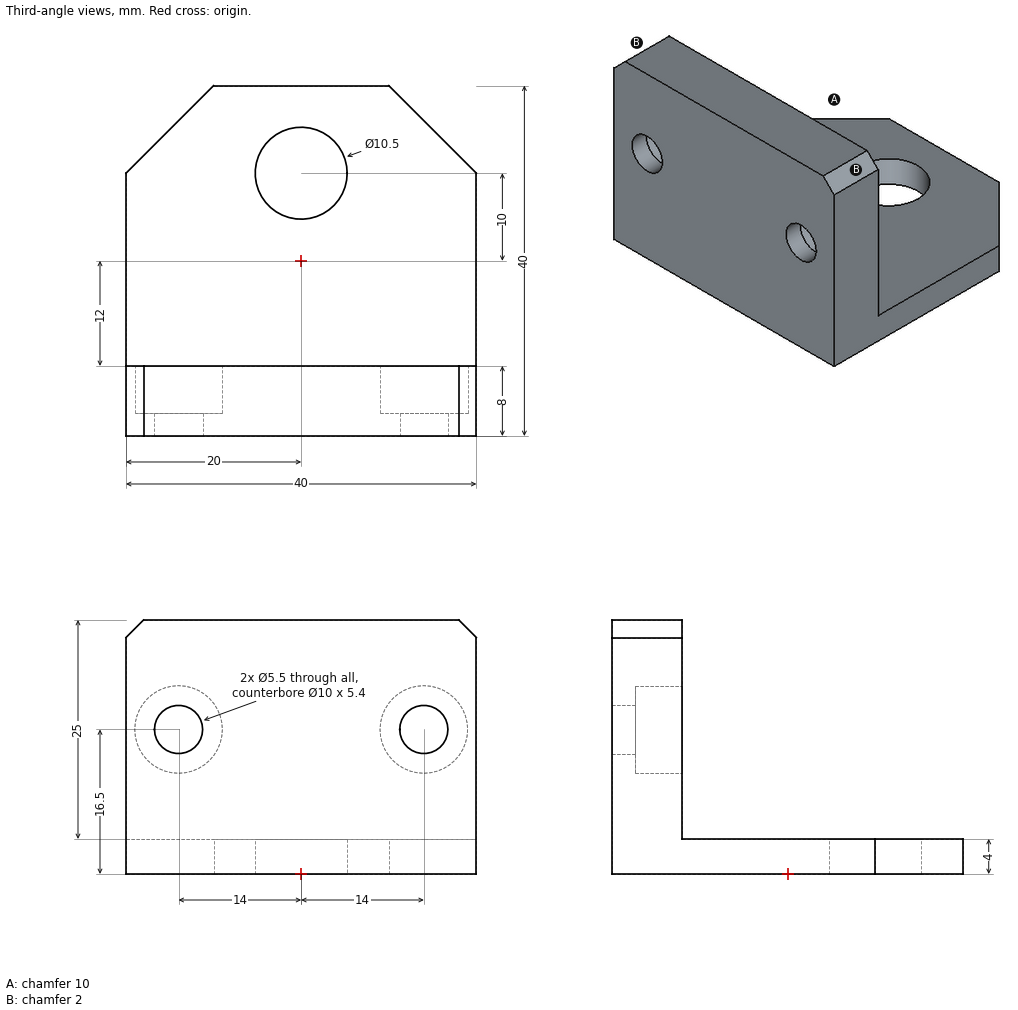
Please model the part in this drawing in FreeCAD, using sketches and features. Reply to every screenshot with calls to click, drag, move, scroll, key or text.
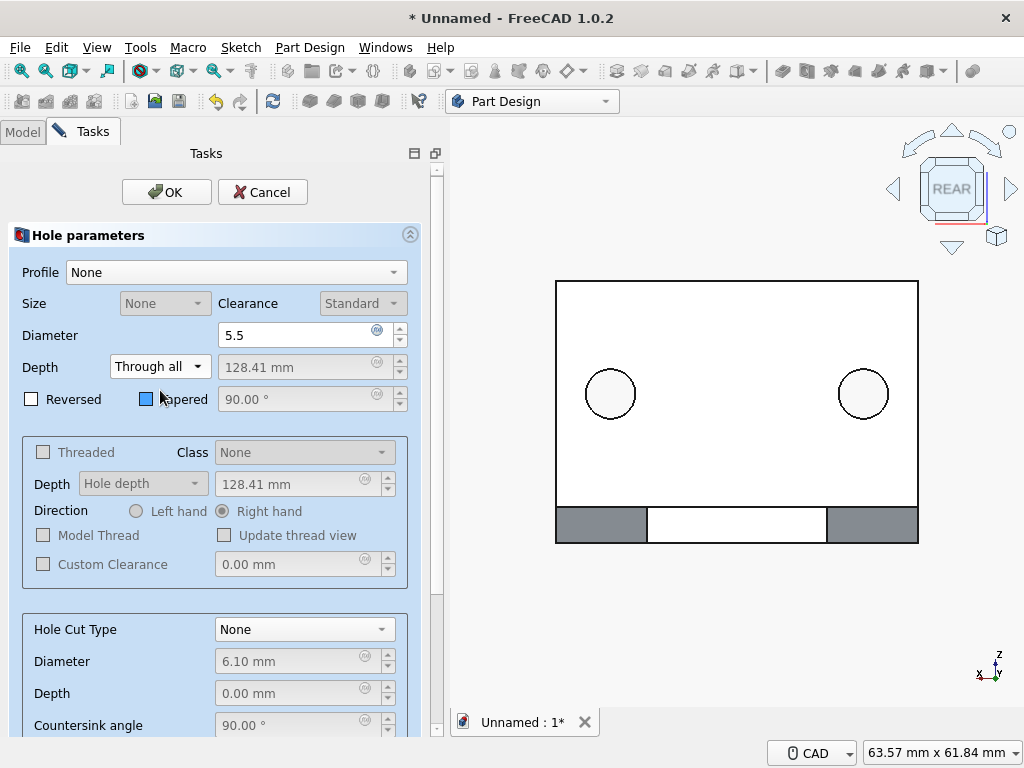
click(306, 630)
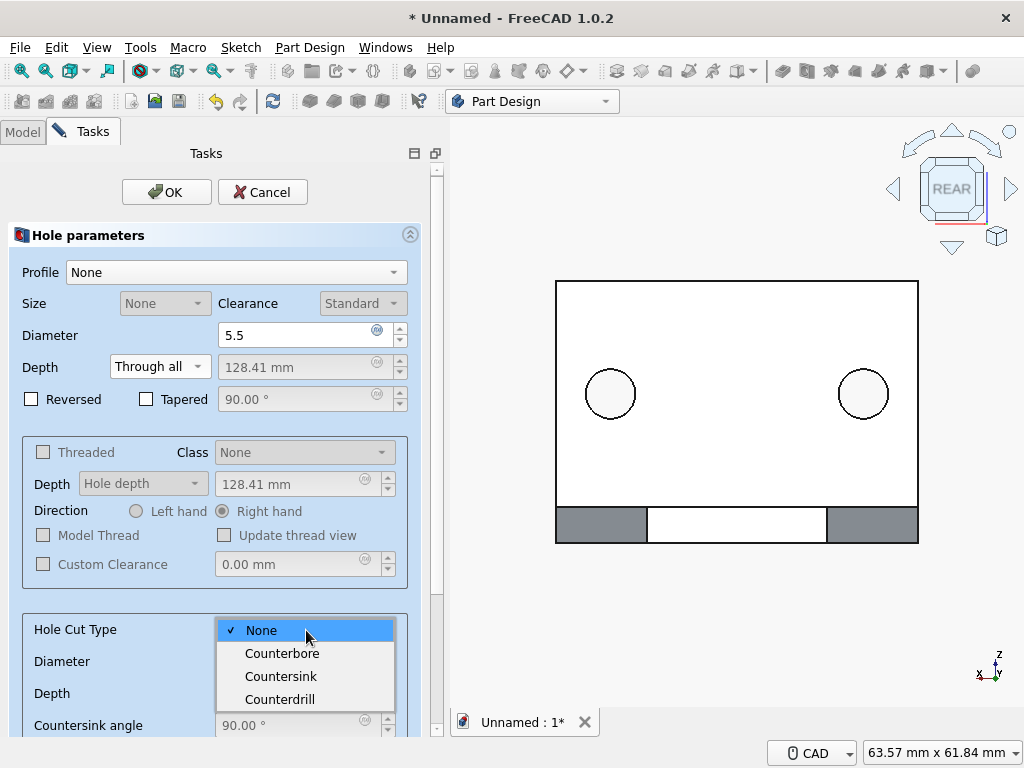
click(304, 654)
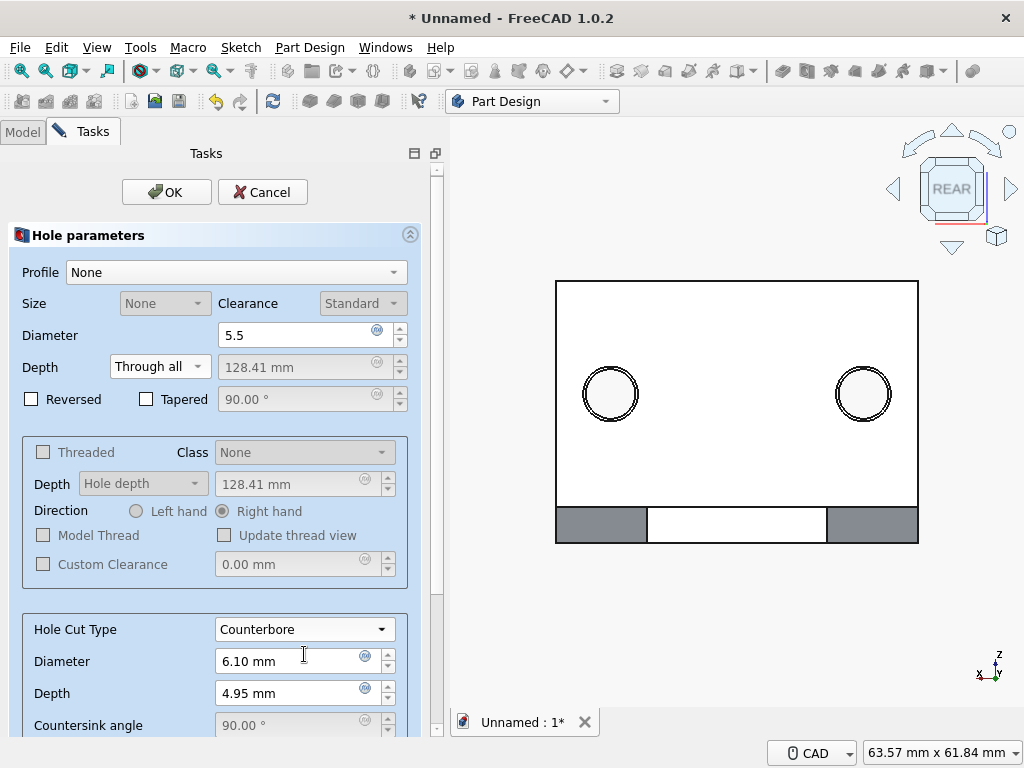
triple_click(298, 661)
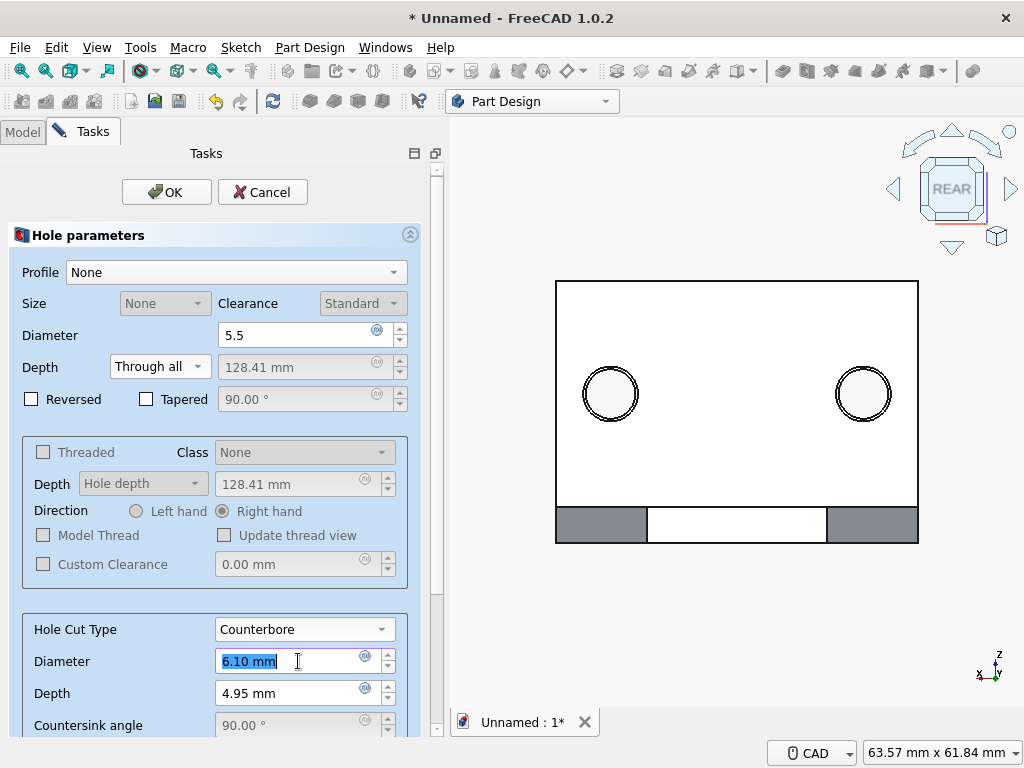
text(10)
key(Tab)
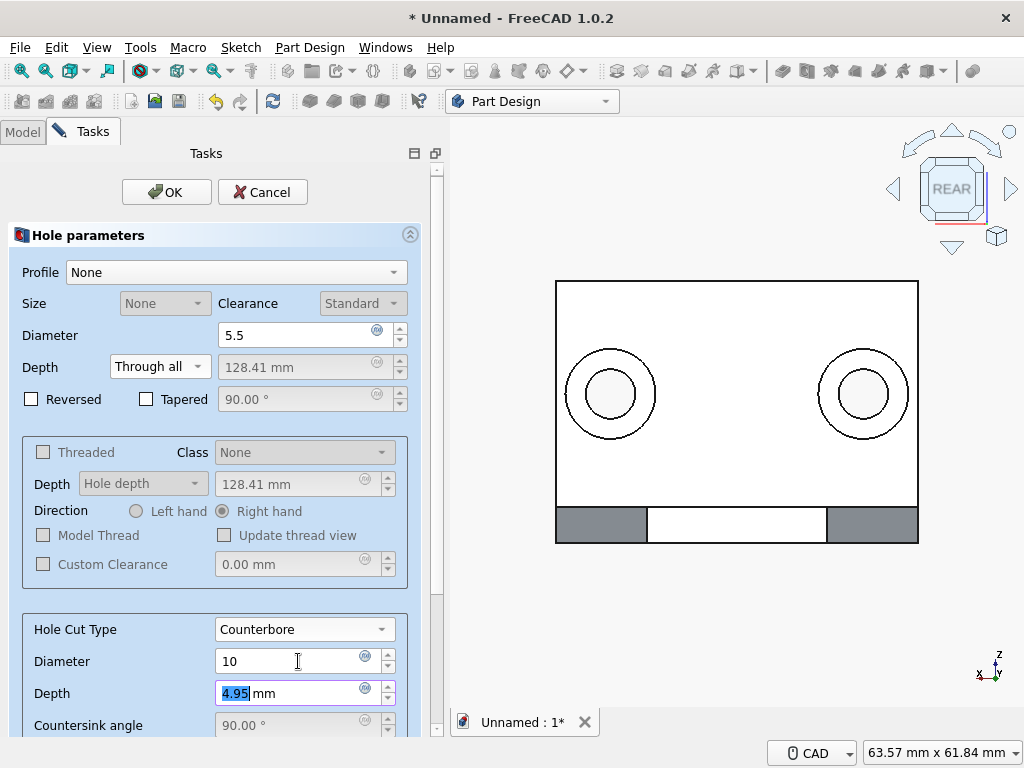
text(5.4)
key(Tab)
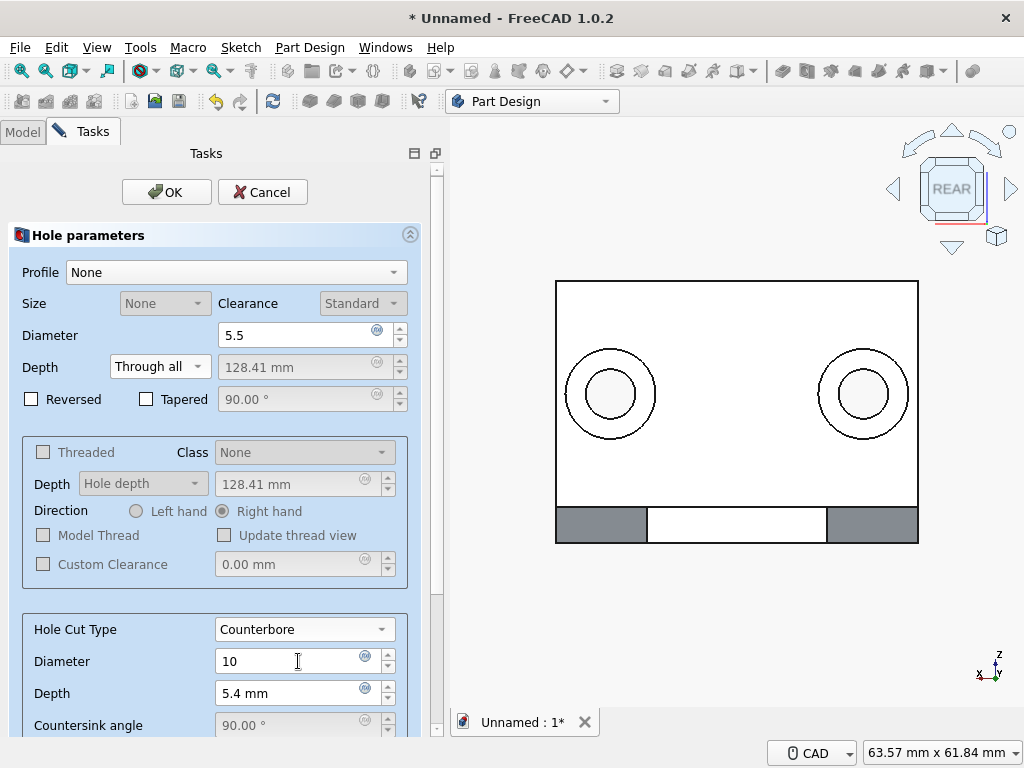
click(167, 192)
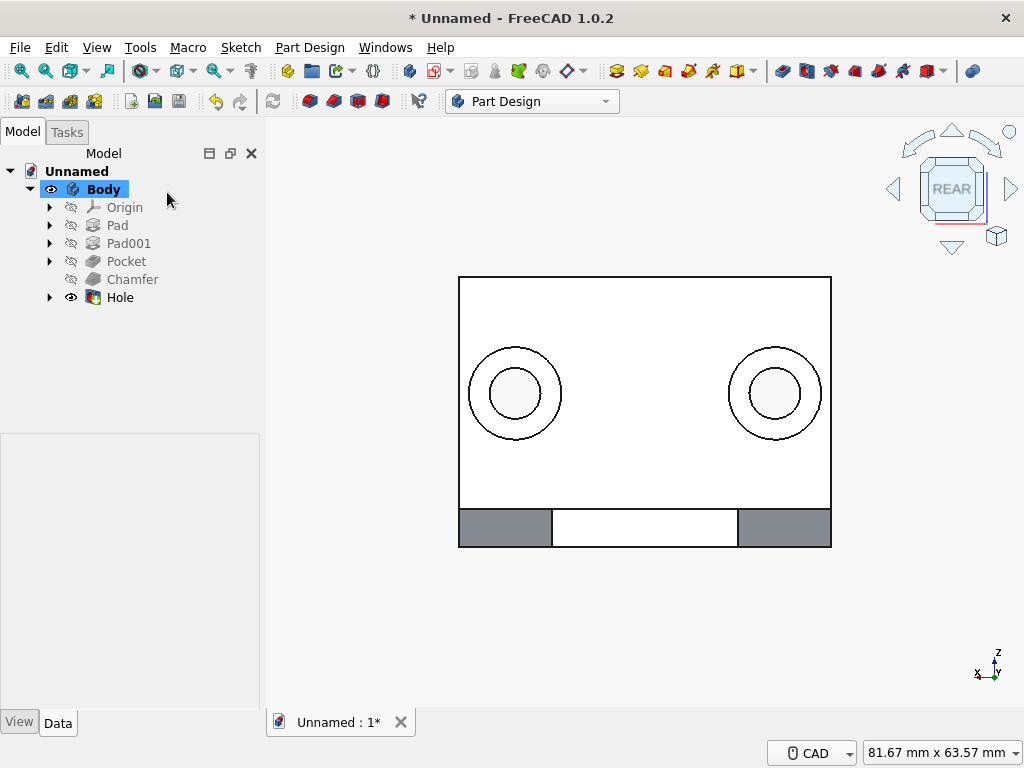
key(0)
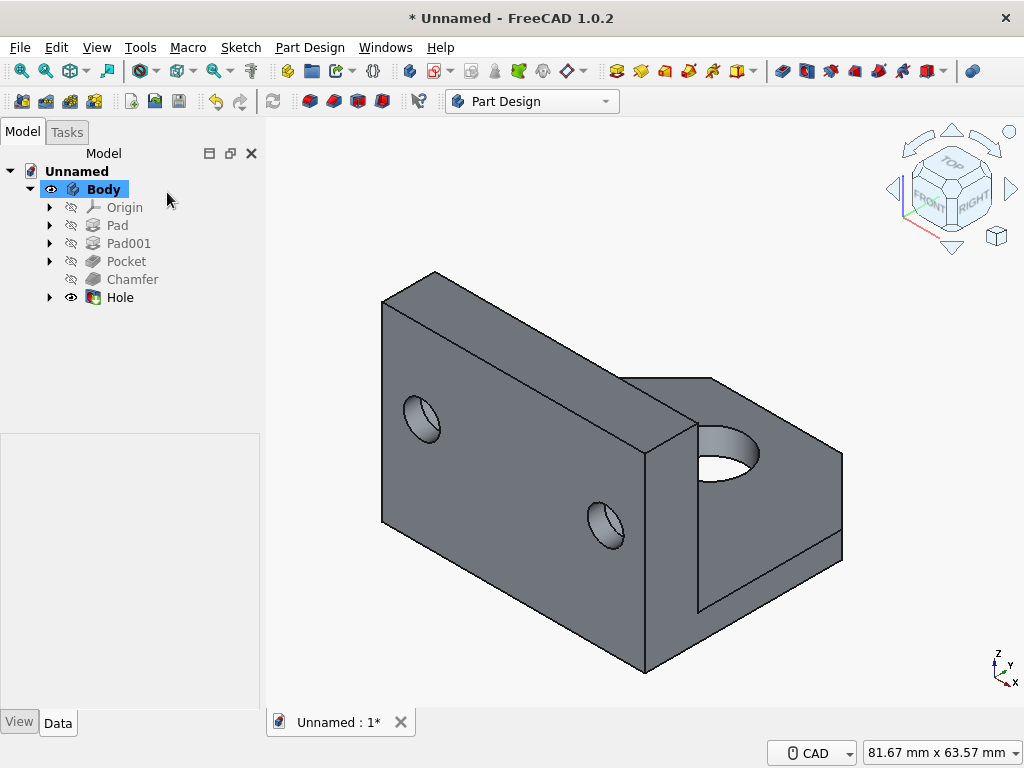
click(671, 438)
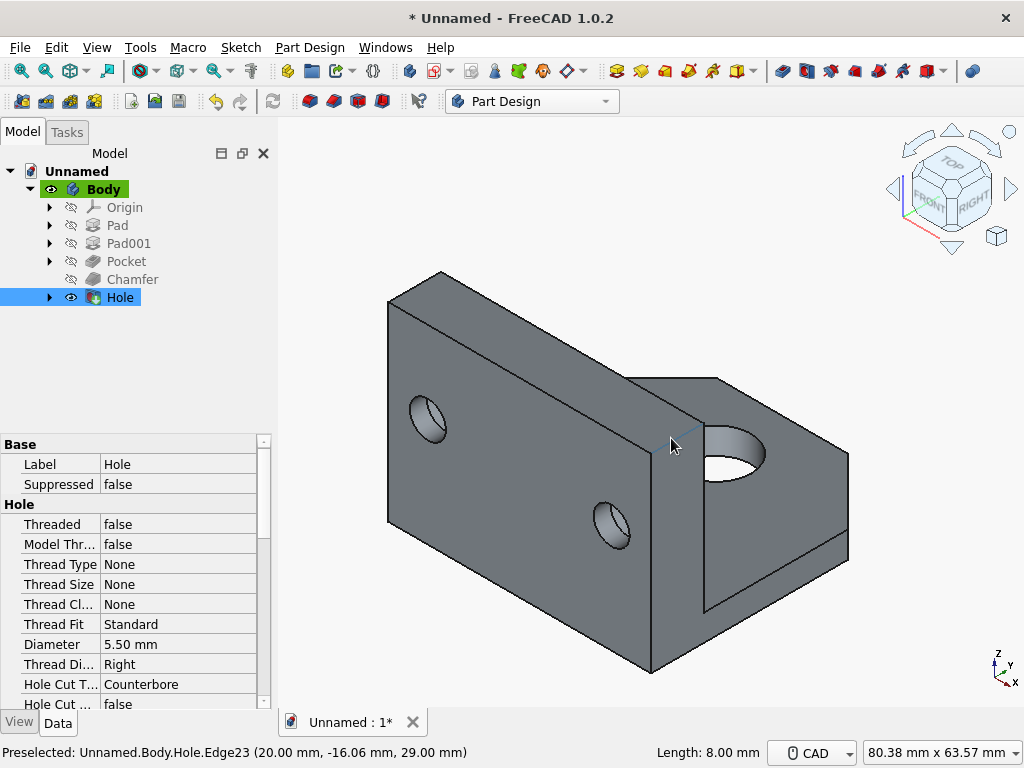
key(2)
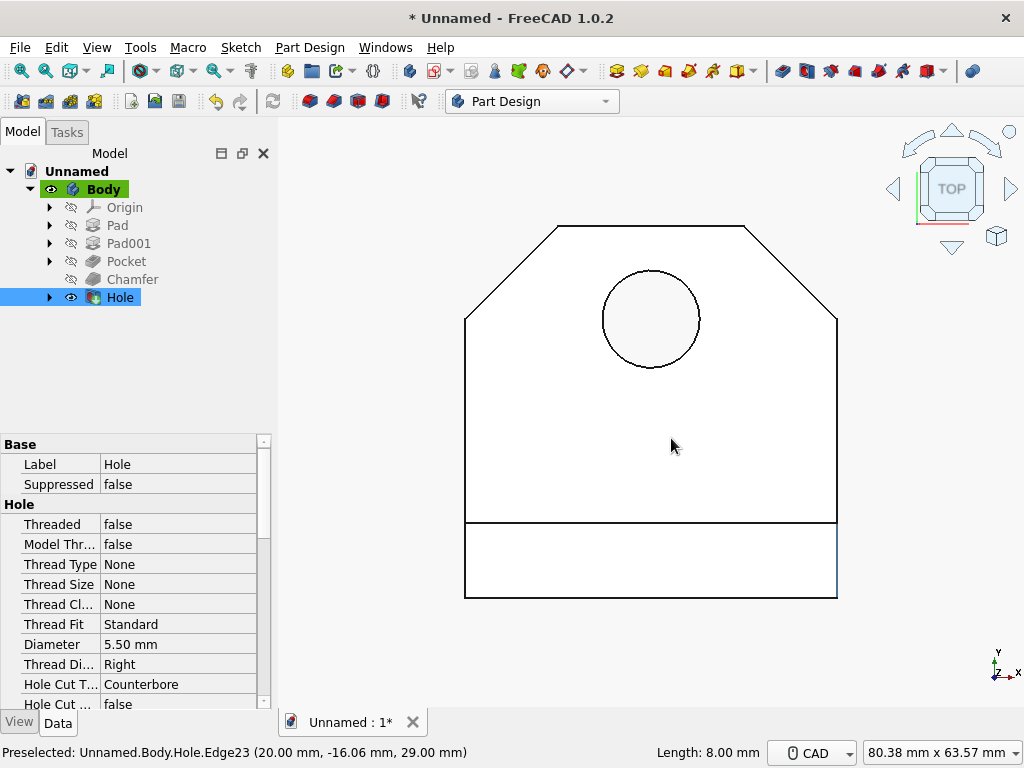
click(465, 560, ctrl)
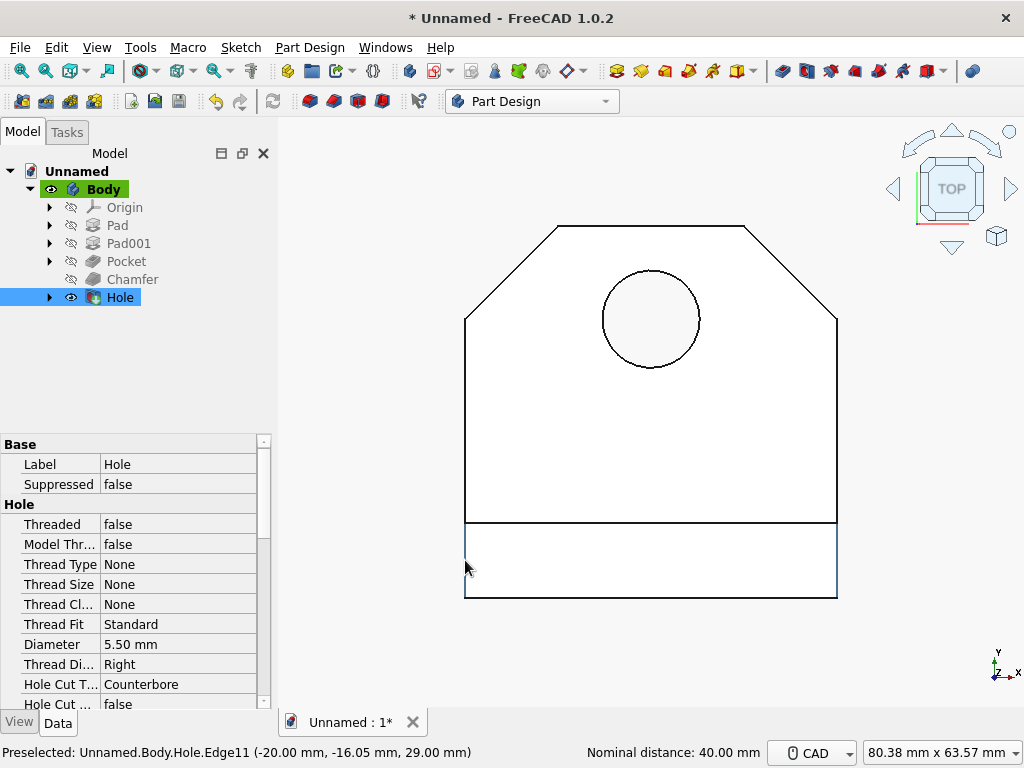
click(334, 102)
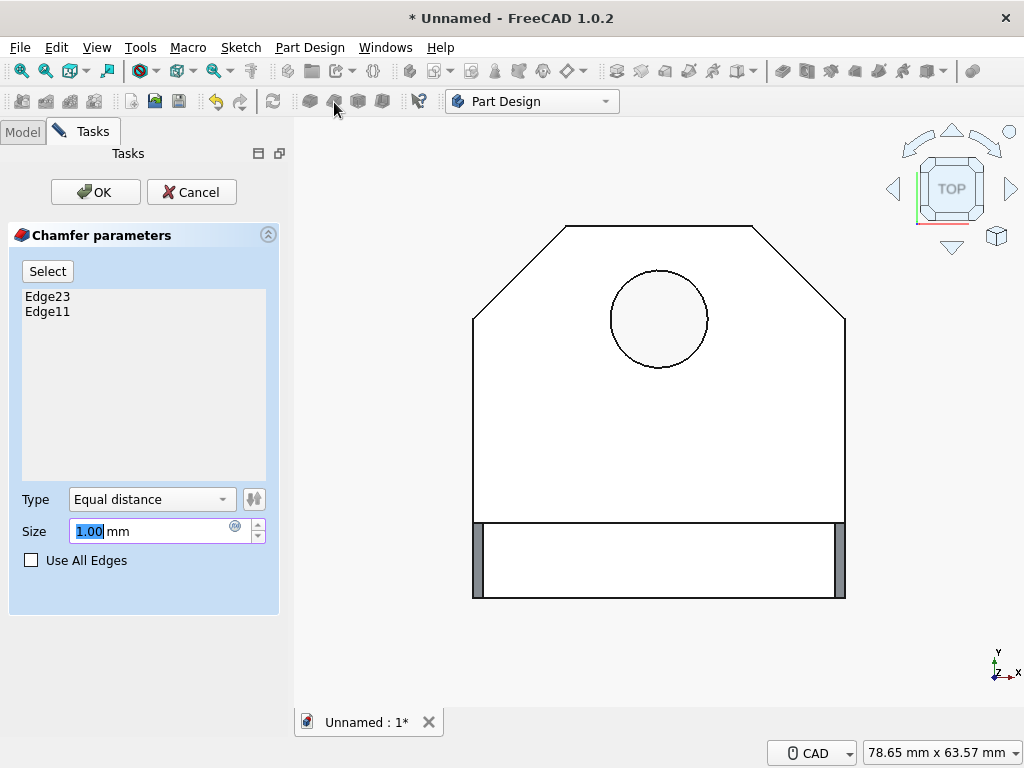
text(2)
key(Tab)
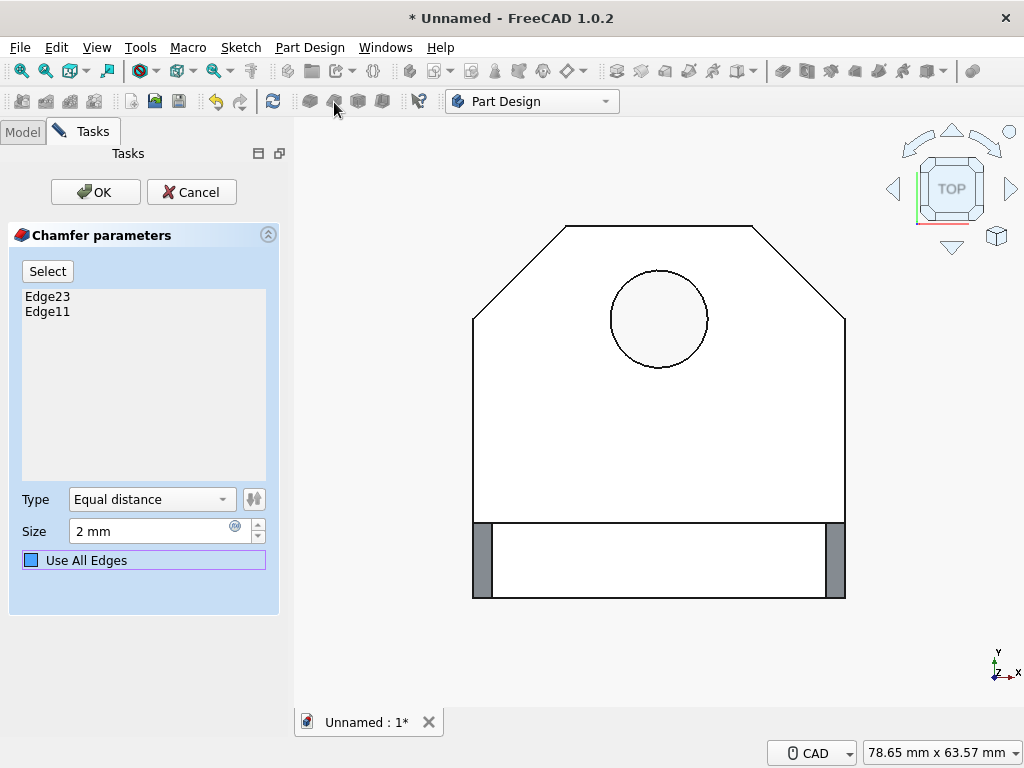
click(96, 192)